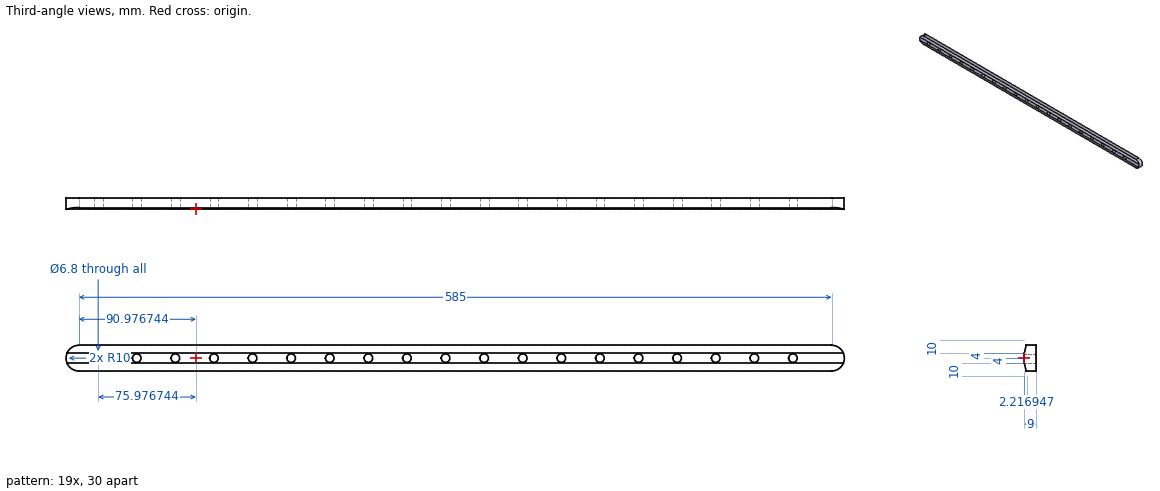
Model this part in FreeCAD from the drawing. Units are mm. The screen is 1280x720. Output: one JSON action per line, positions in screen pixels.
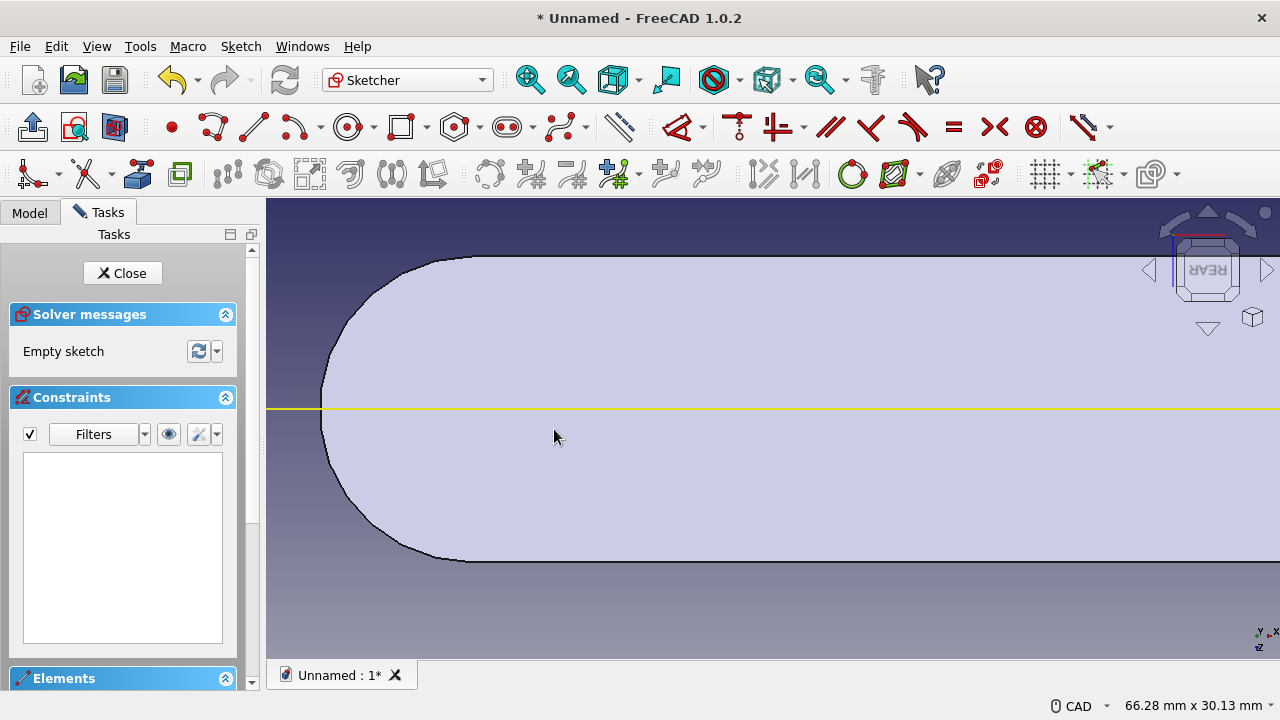
{"action": "scroll", "coordinate": [701, 398], "scroll_direction": "up", "scroll_amount": 5}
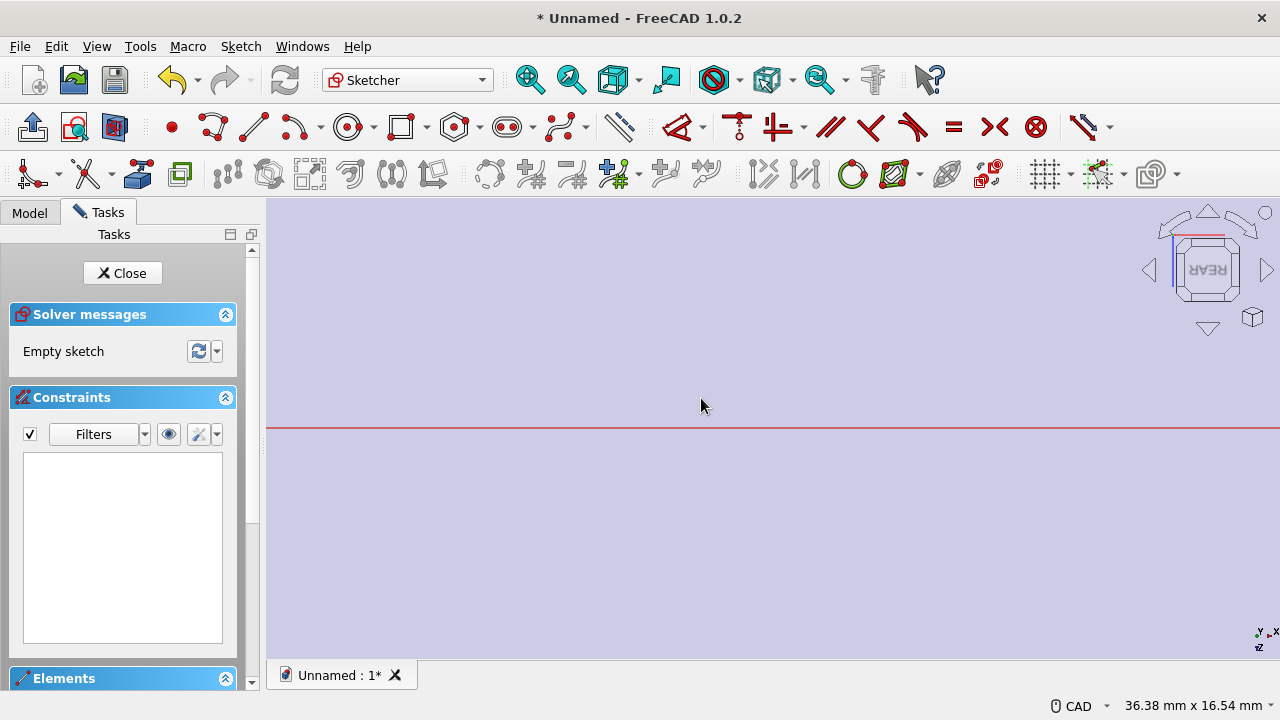
{"action": "left_click", "coordinate": [348, 128]}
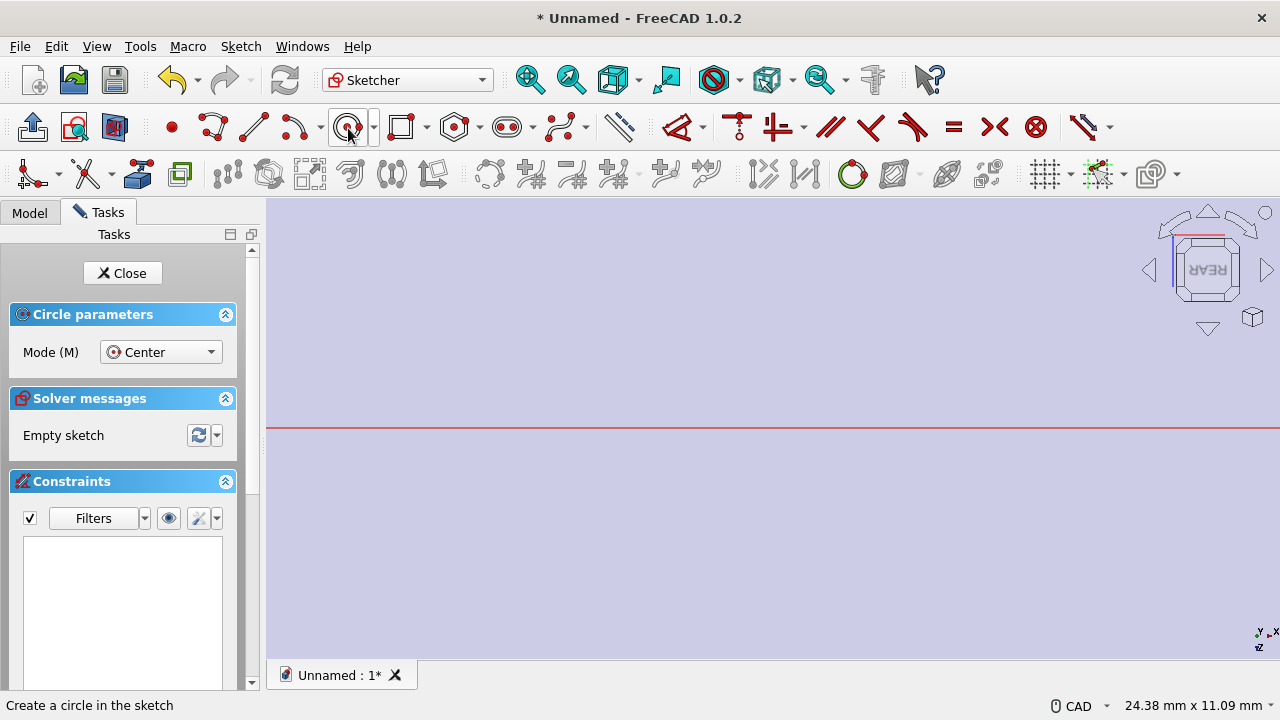
{"action": "left_click", "coordinate": [703, 428]}
{"action": "mouse_move", "coordinate": [803, 328]}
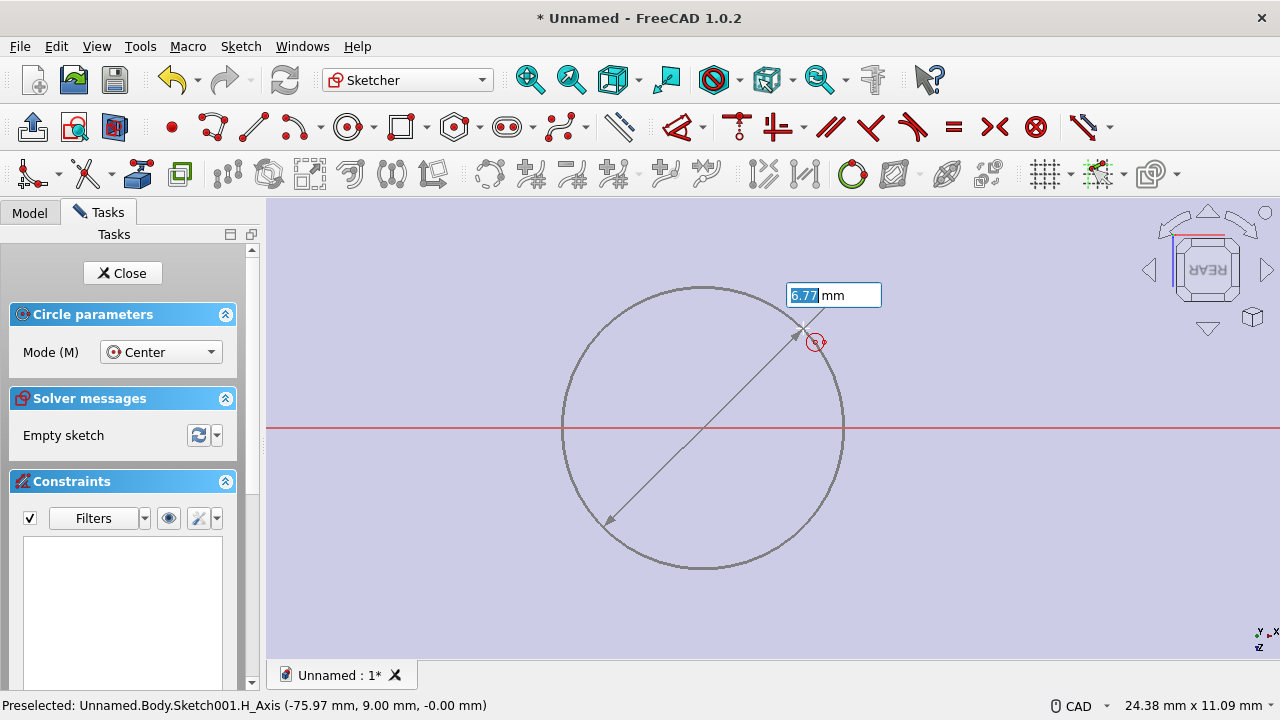
{"action": "type", "text": "6.8"}
{"action": "key", "text": "Return"}
{"action": "key", "text": "Escape"}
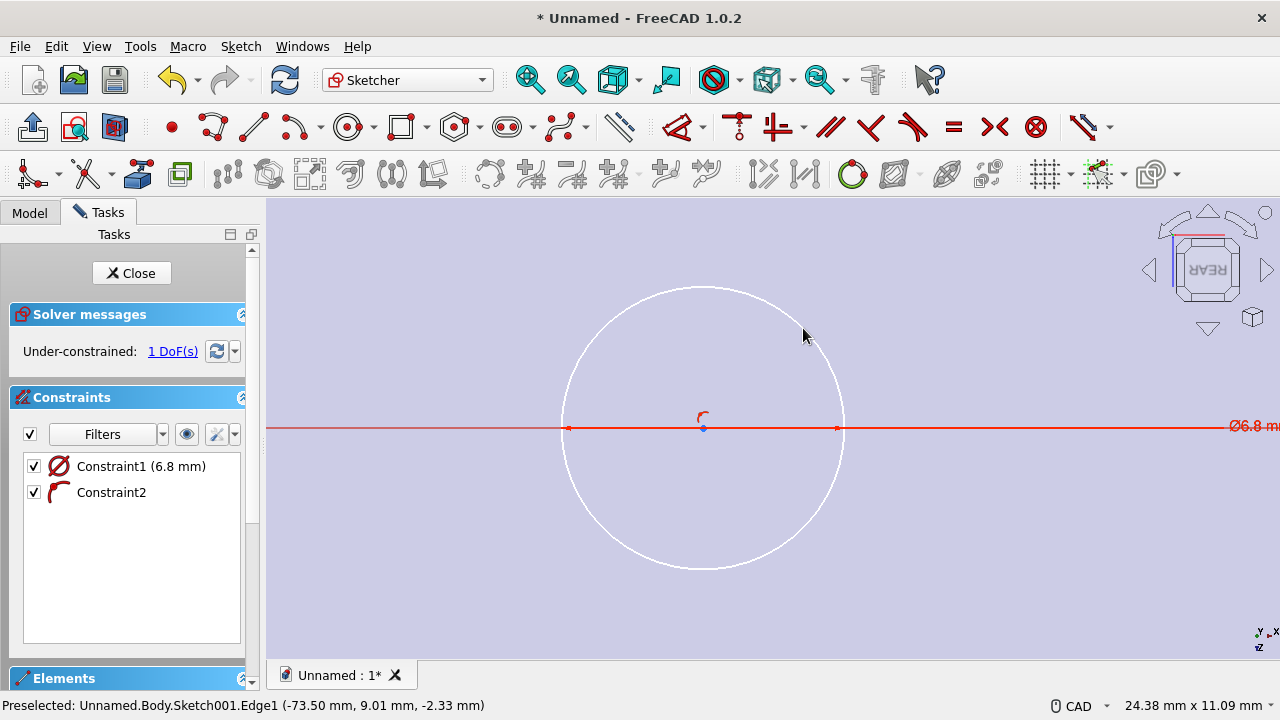
{"action": "left_click", "coordinate": [676, 128]}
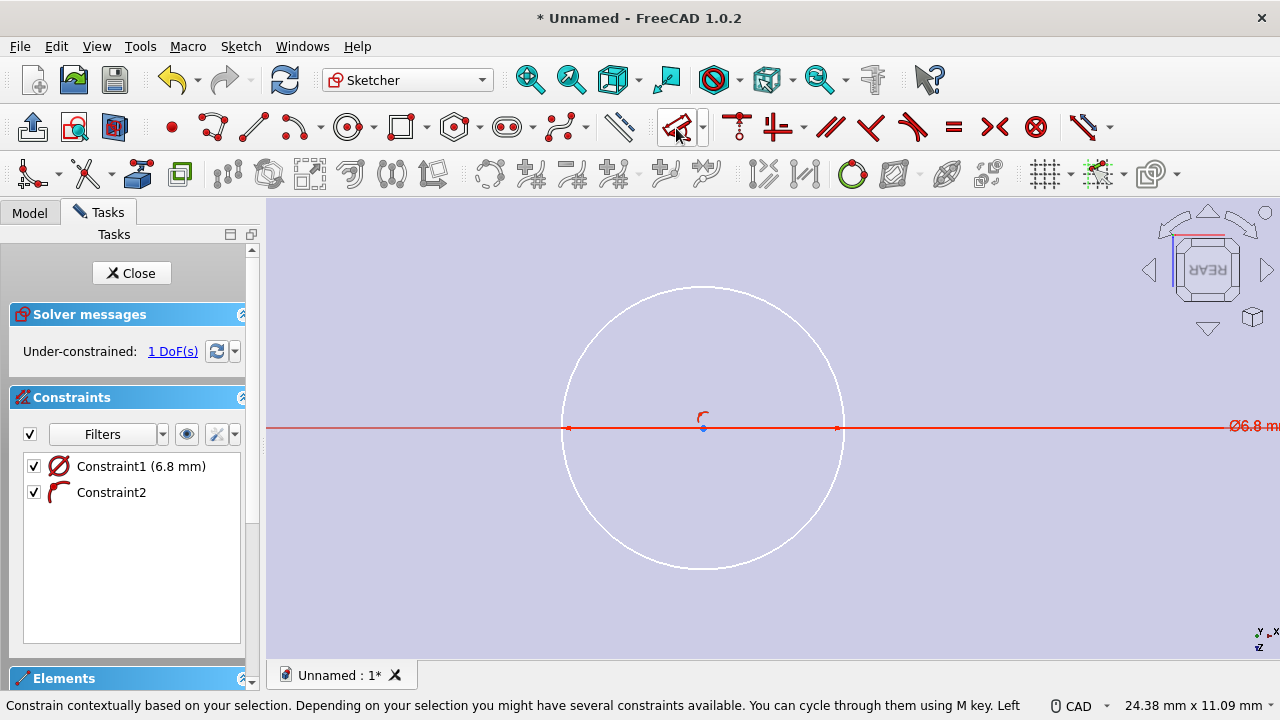
{"action": "left_click", "coordinate": [703, 428]}
{"action": "left_click", "coordinate": [909, 462]}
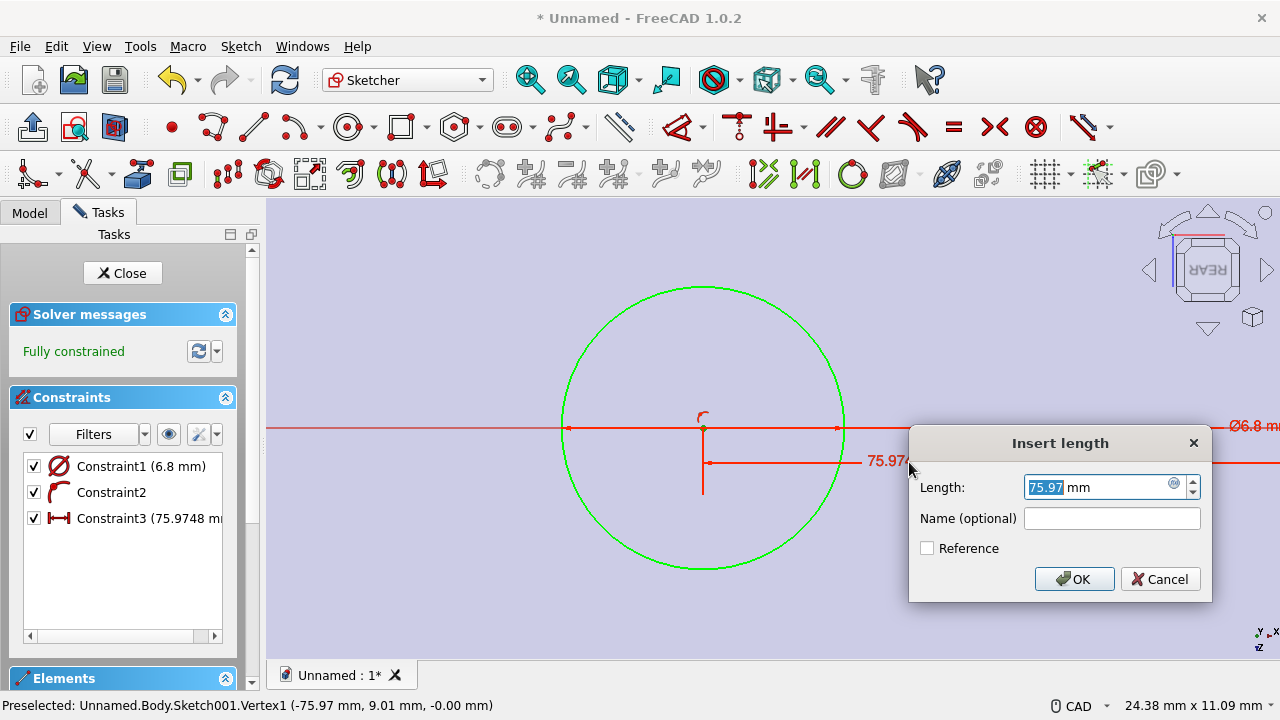
{"action": "type", "text": "75.976744"}
{"action": "key", "text": "Return"}
{"action": "key", "text": "Escape"}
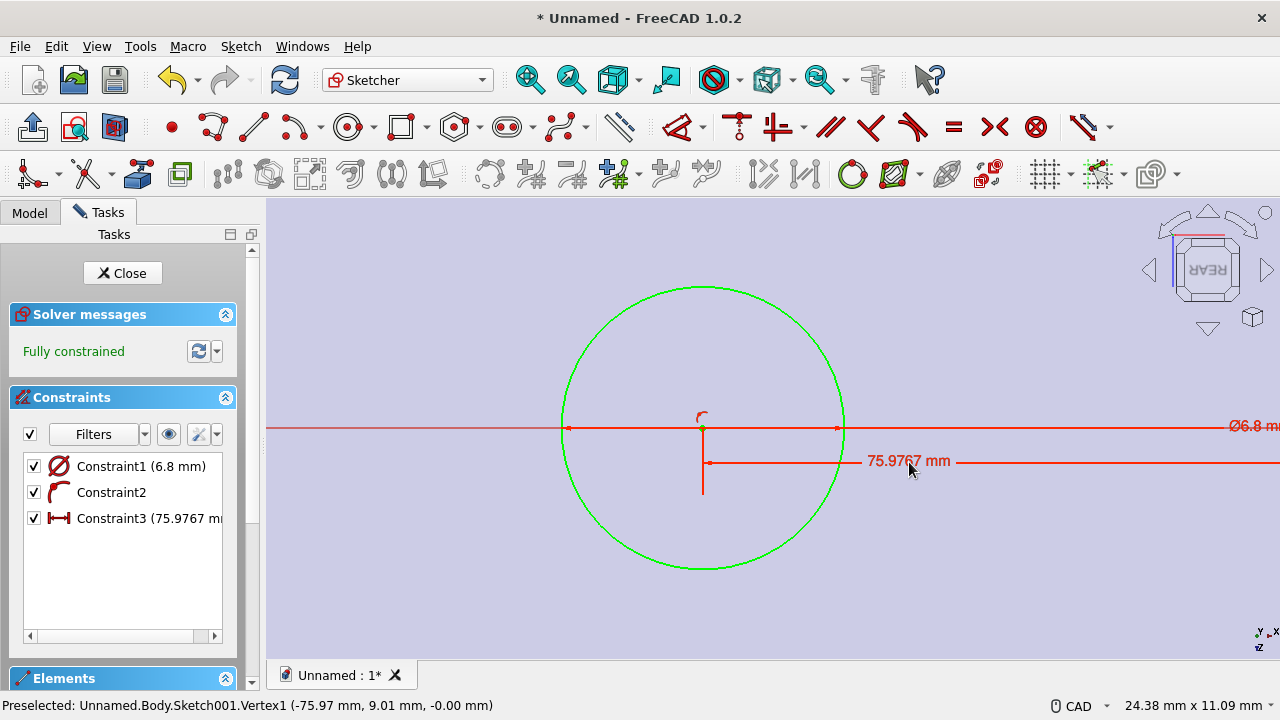
{"action": "left_click", "coordinate": [123, 273]}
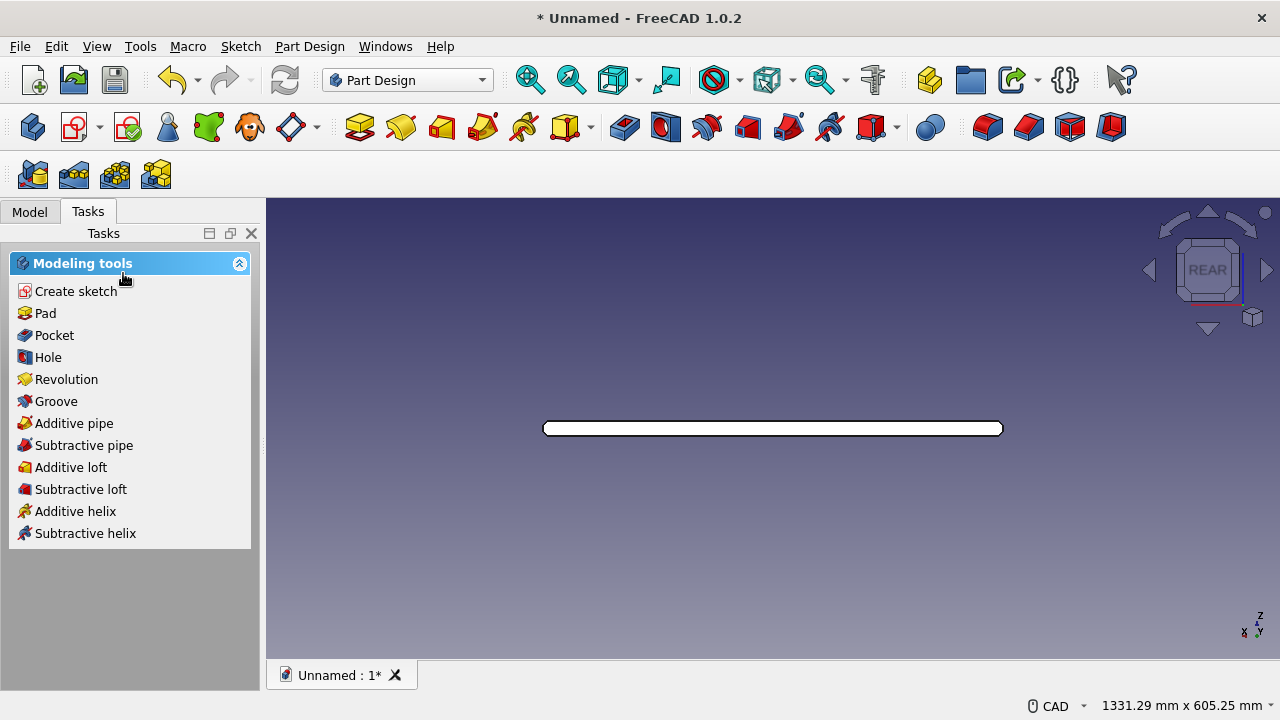
{"action": "left_click", "coordinate": [666, 128]}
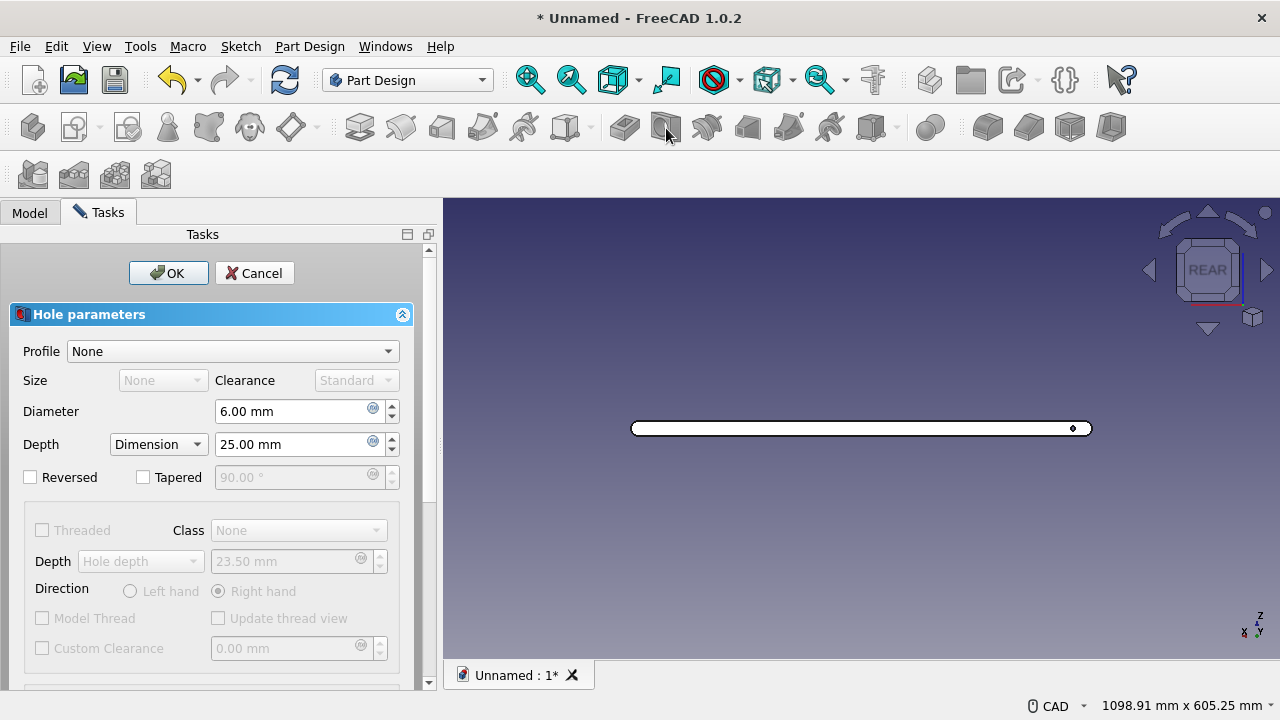
{"action": "triple_click", "coordinate": [300, 412]}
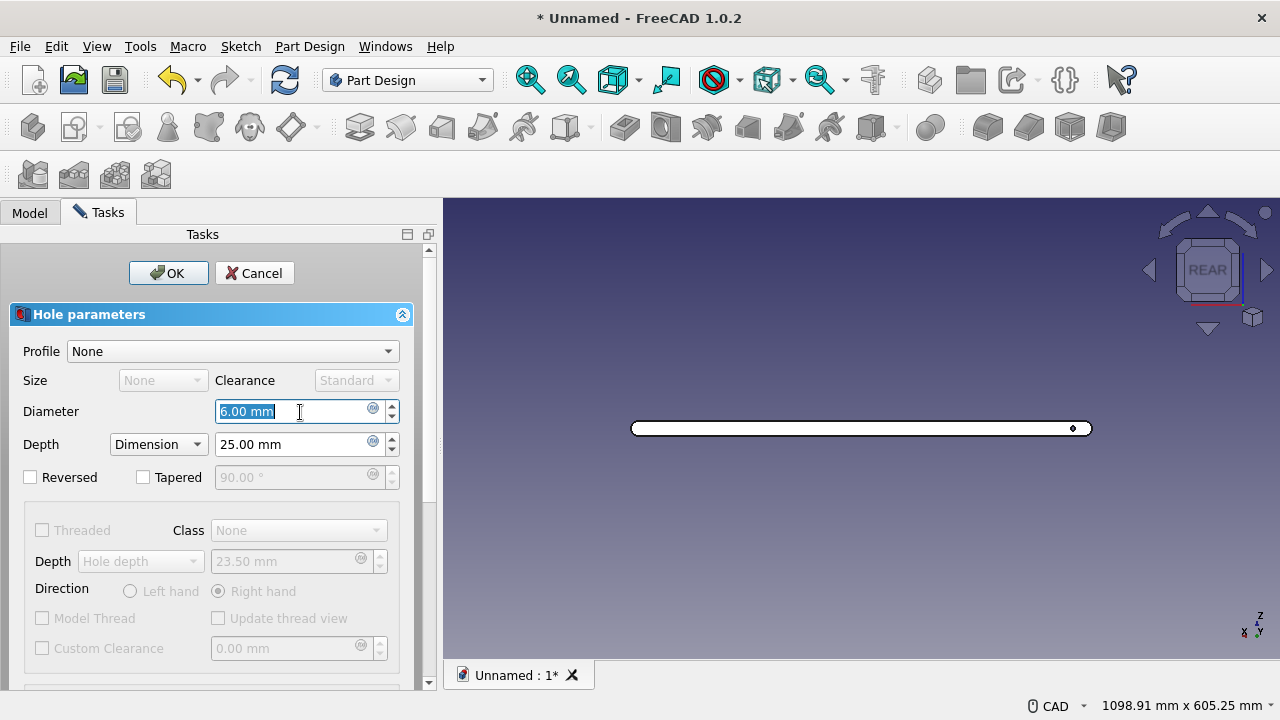
{"action": "type", "text": "6.8"}
{"action": "key", "text": "Tab"}